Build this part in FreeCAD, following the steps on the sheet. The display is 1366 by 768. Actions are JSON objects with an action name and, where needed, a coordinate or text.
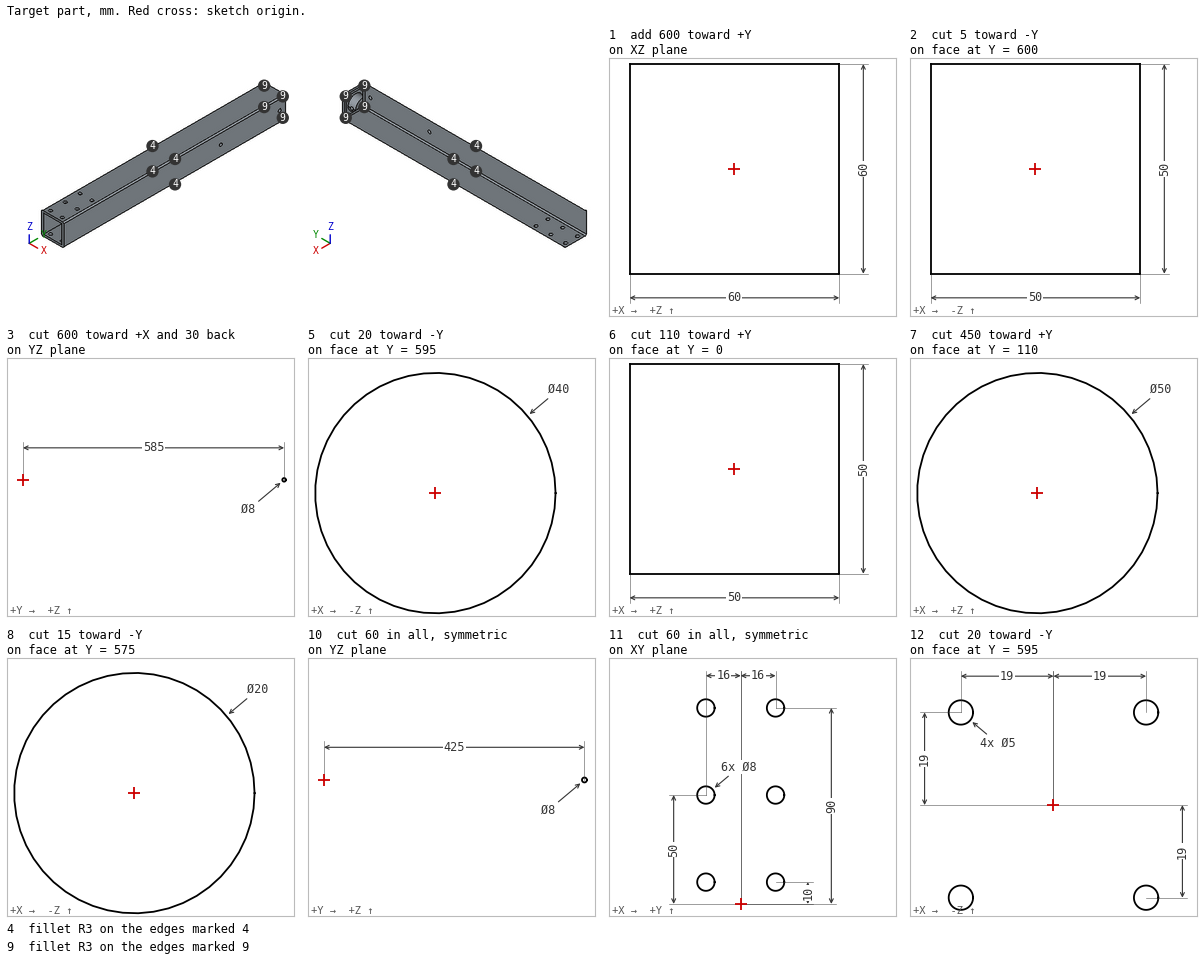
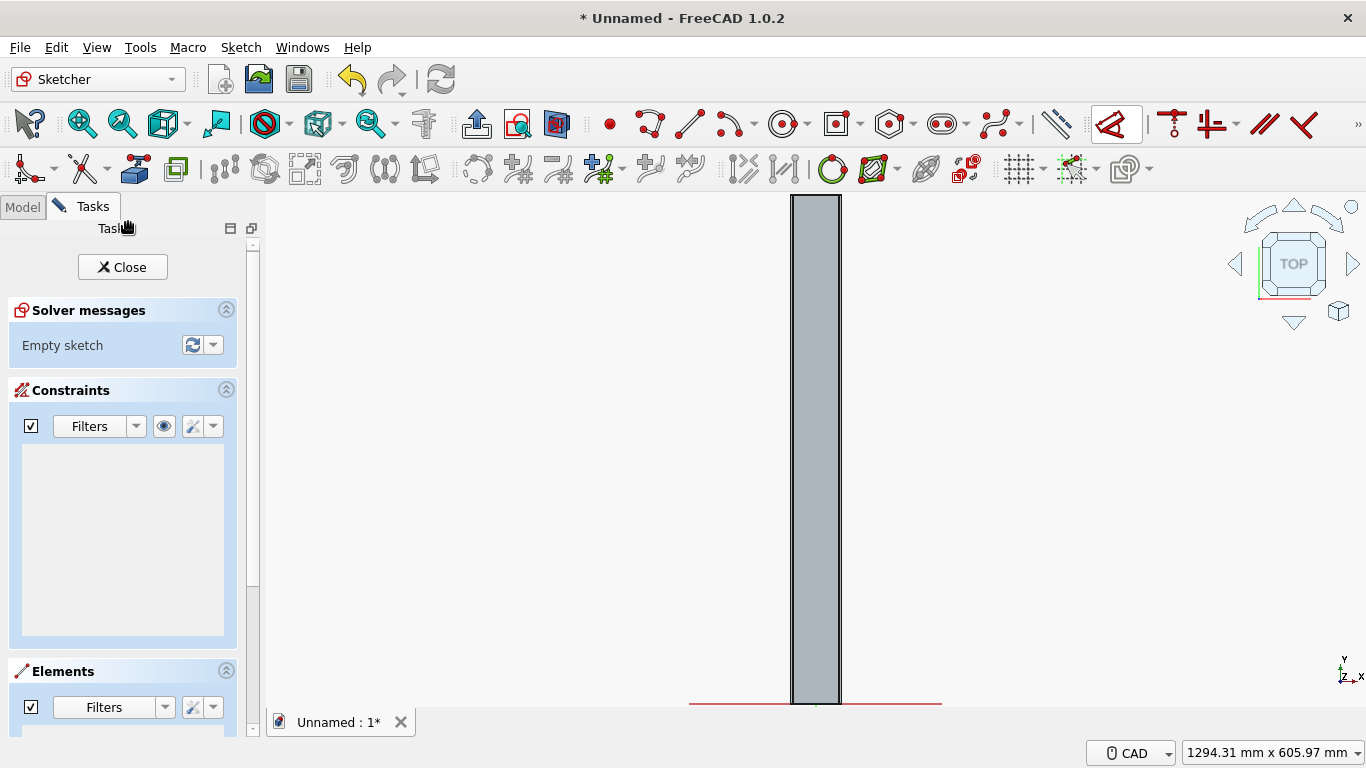
{"action": "left_click", "coordinate": [558, 124]}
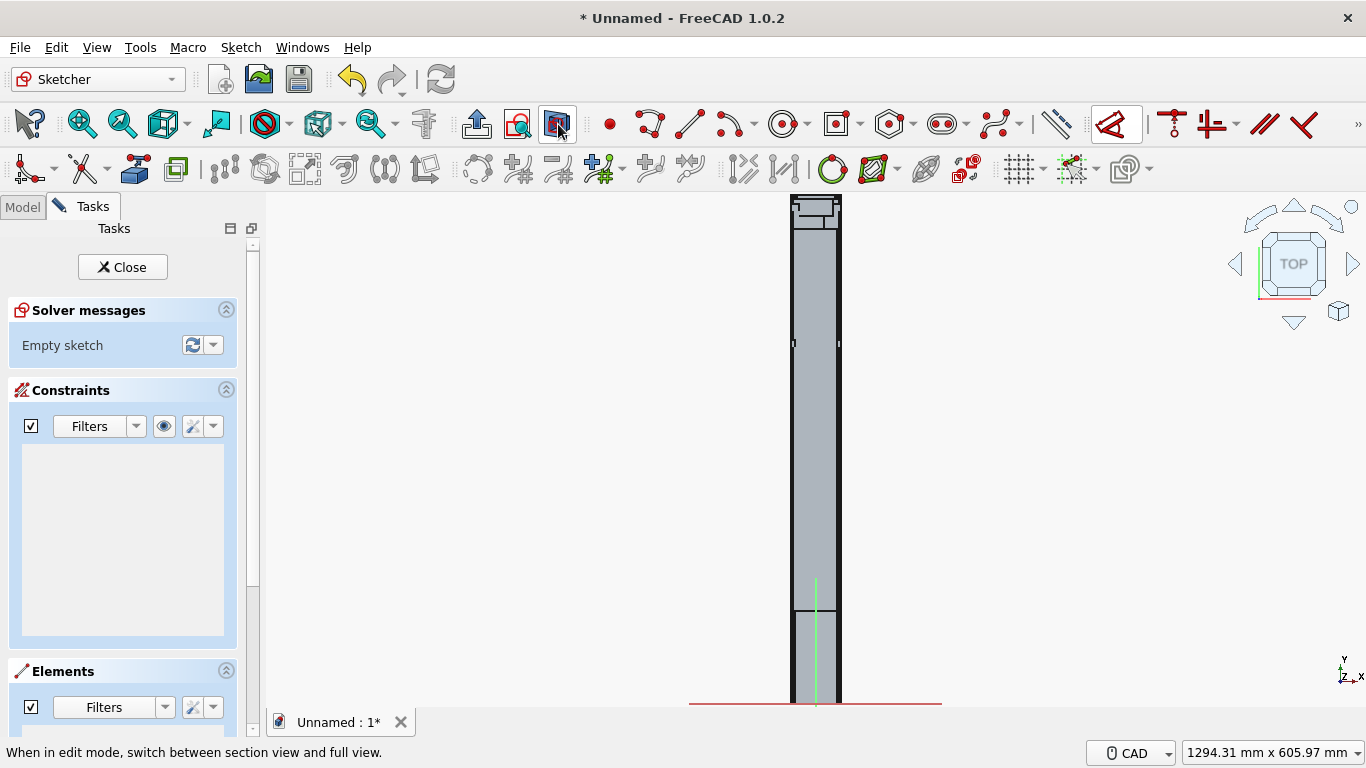
{"action": "scroll", "coordinate": [748, 450], "scroll_direction": "down", "scroll_amount": 5}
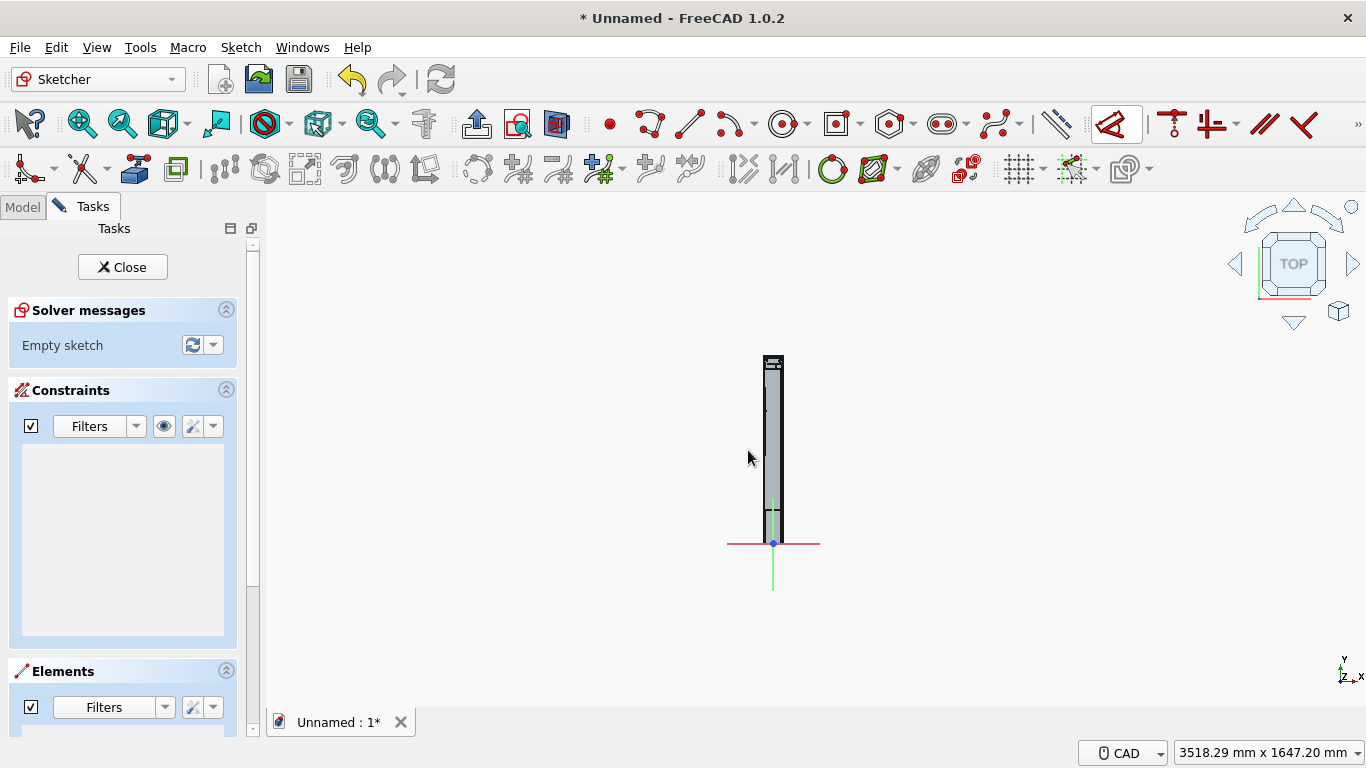
{"action": "scroll", "coordinate": [776, 537], "scroll_direction": "up", "scroll_amount": 12}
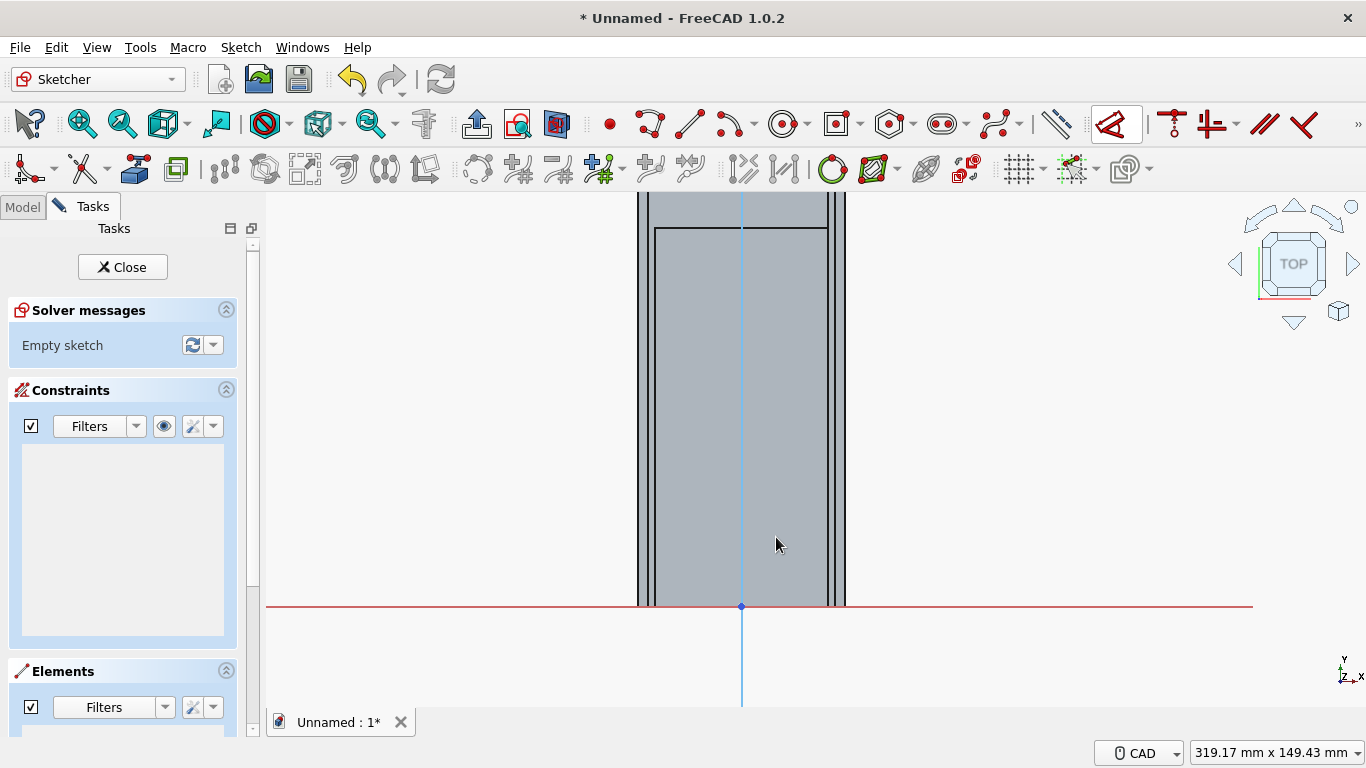
{"action": "left_click", "coordinate": [784, 124]}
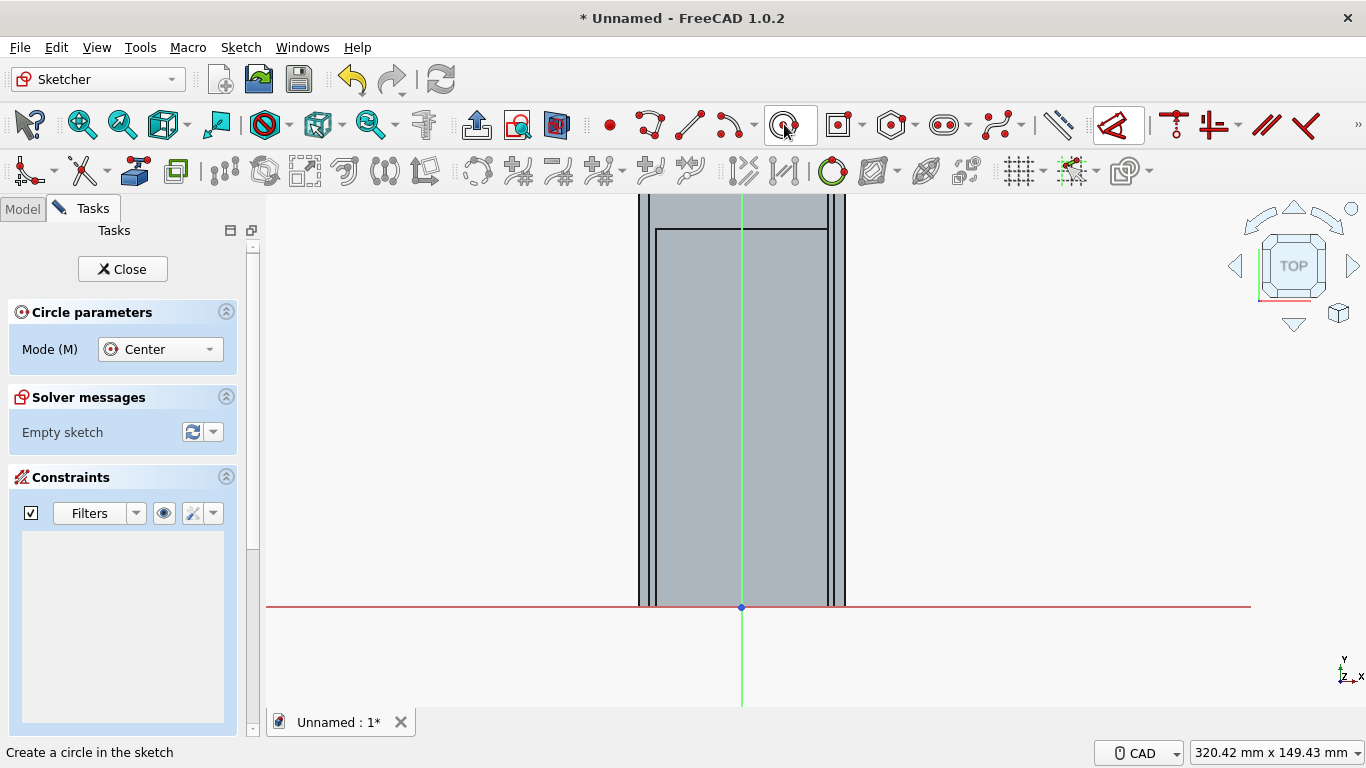
{"action": "scroll", "coordinate": [687, 435], "scroll_direction": "up", "scroll_amount": 3}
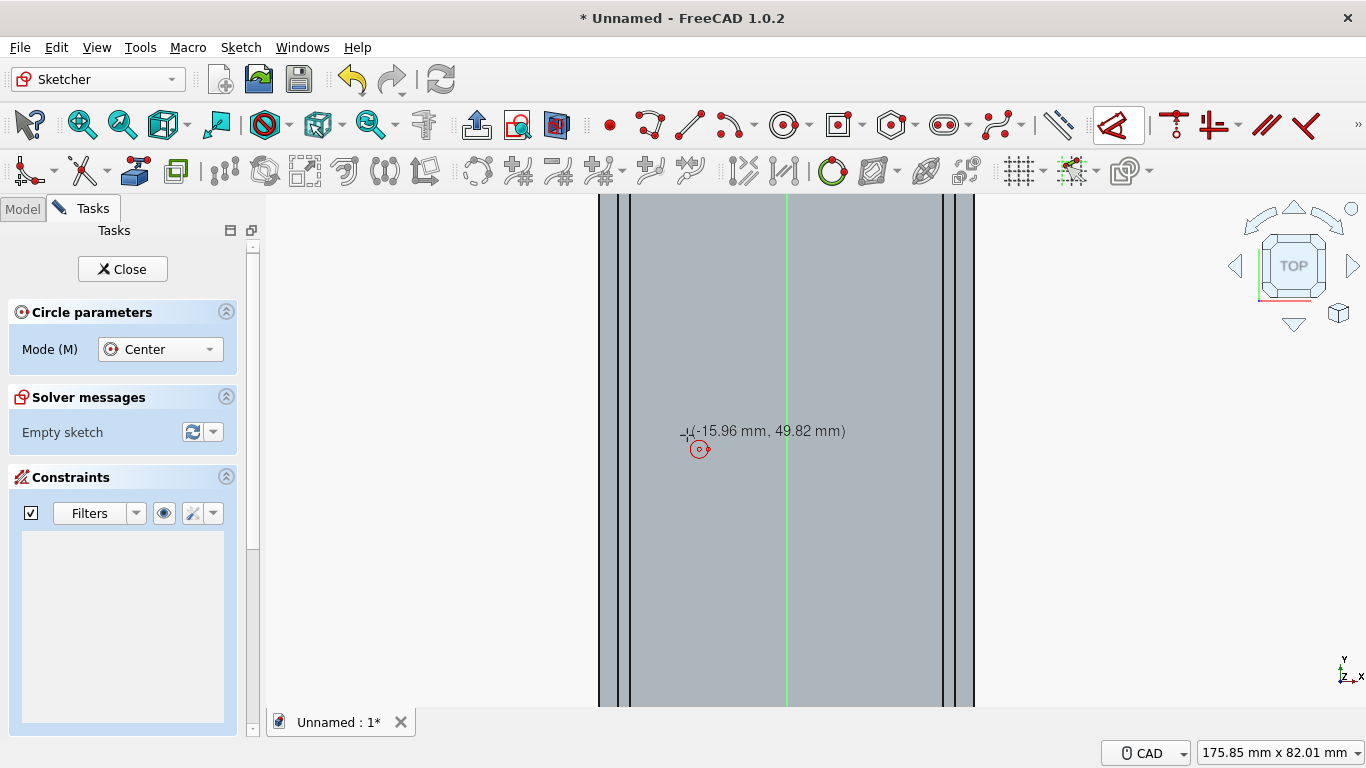
{"action": "left_click", "coordinate": [686, 435]}
{"action": "mouse_move", "coordinate": [704, 418]}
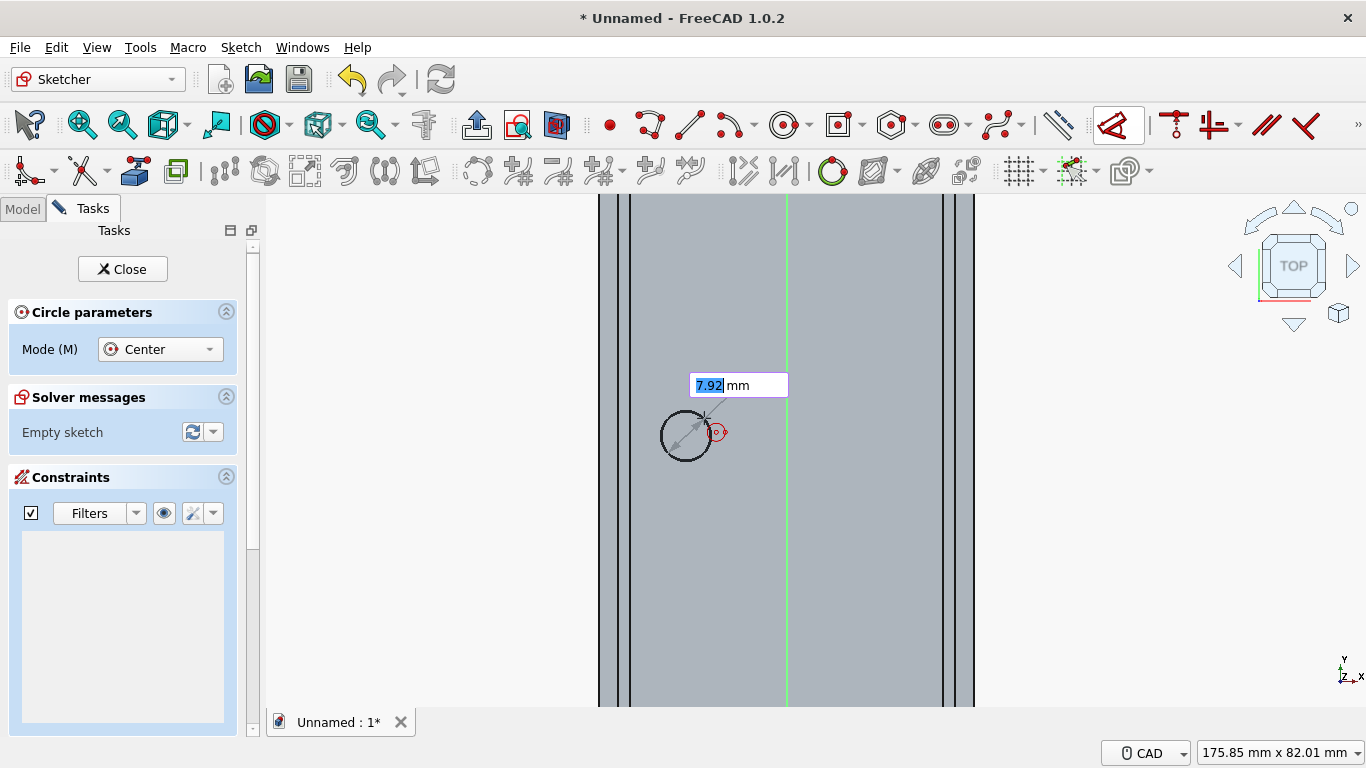
{"action": "type", "text": "8"}
{"action": "key", "text": "Return"}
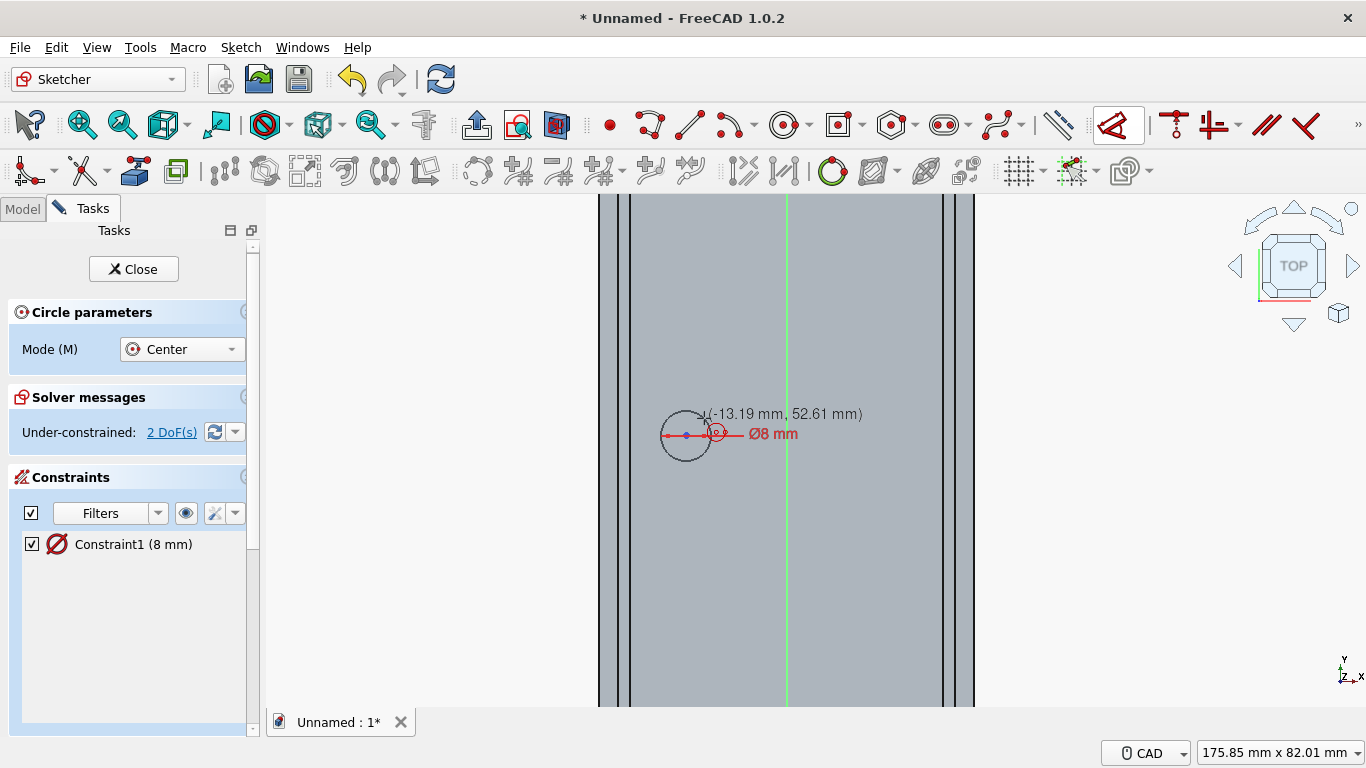
{"action": "scroll", "coordinate": [700, 446], "scroll_direction": "down", "scroll_amount": 3}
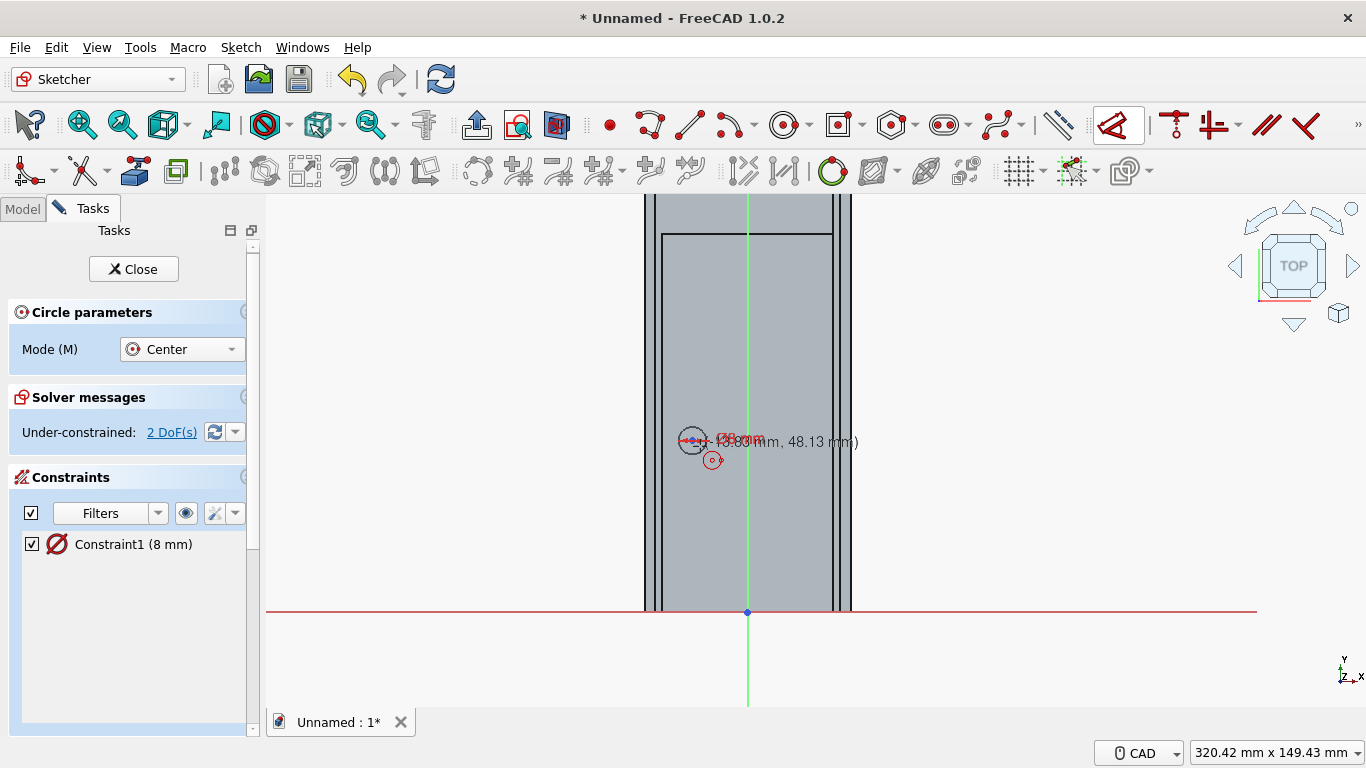
{"action": "scroll", "coordinate": [803, 303], "scroll_direction": "up", "scroll_amount": 3}